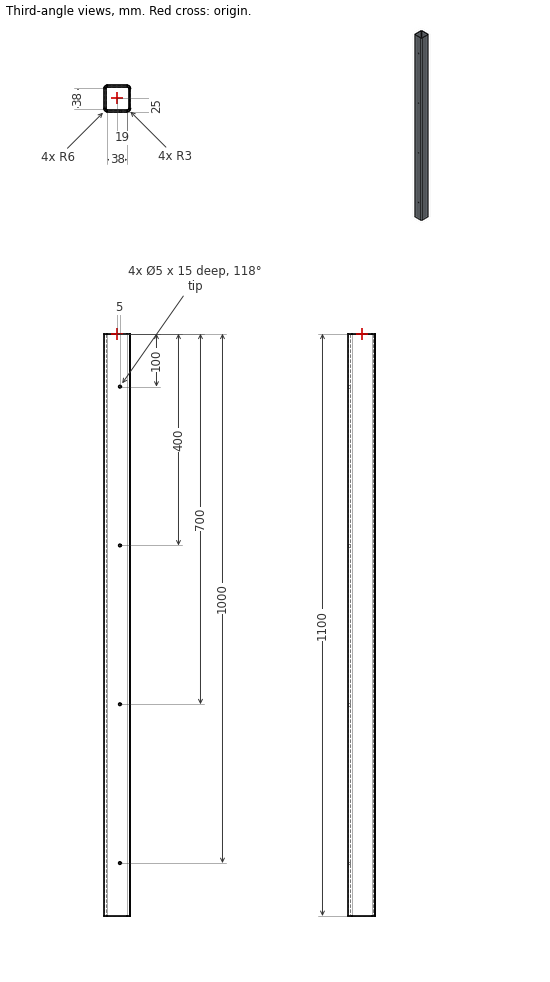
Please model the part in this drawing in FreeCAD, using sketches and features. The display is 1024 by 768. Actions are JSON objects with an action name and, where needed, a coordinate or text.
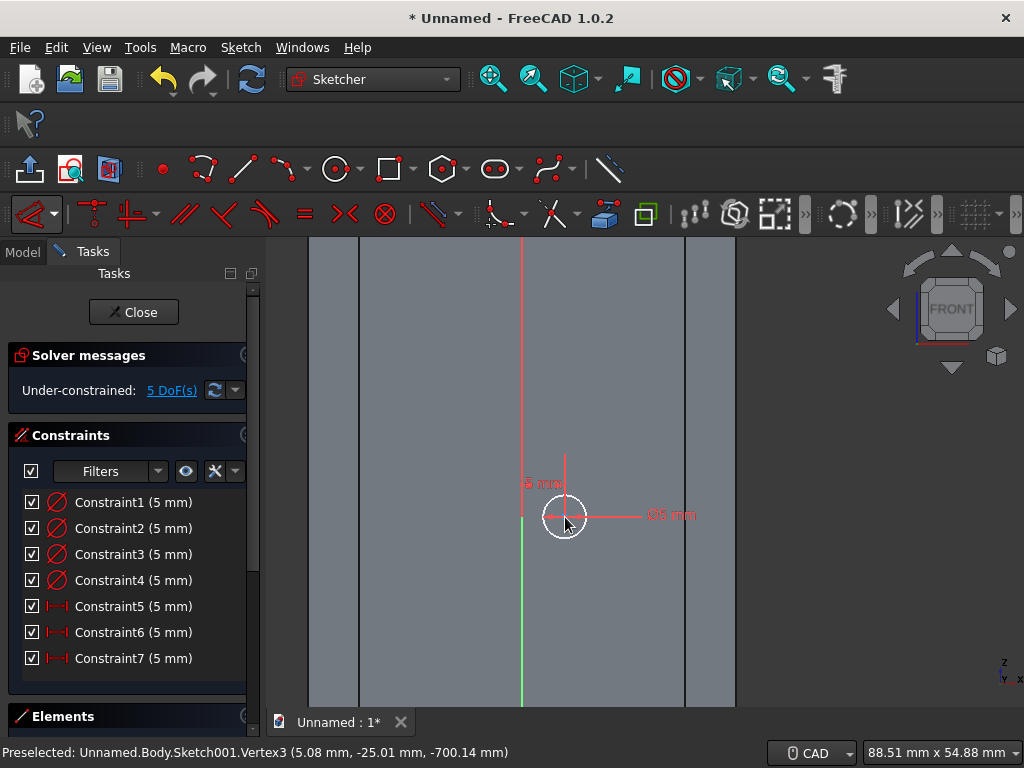
{"action": "scroll", "coordinate": [577, 542], "scroll_direction": "down", "scroll_amount": 16}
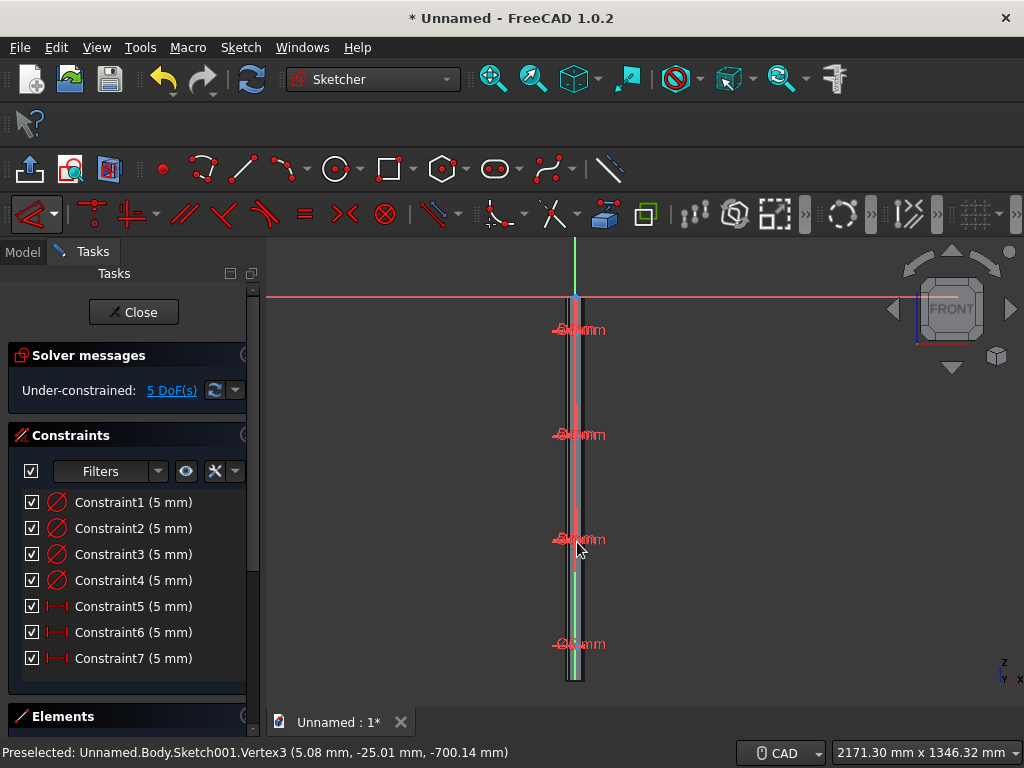
{"action": "scroll", "coordinate": [577, 646], "scroll_direction": "up", "scroll_amount": 16}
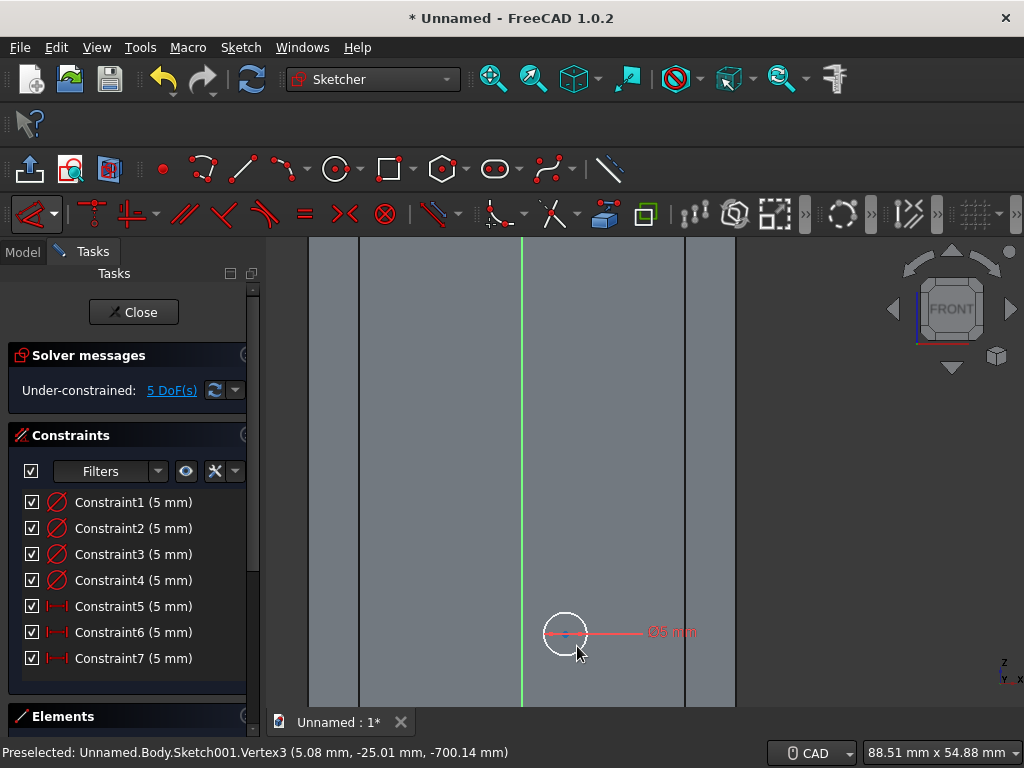
{"action": "left_click", "coordinate": [565, 634]}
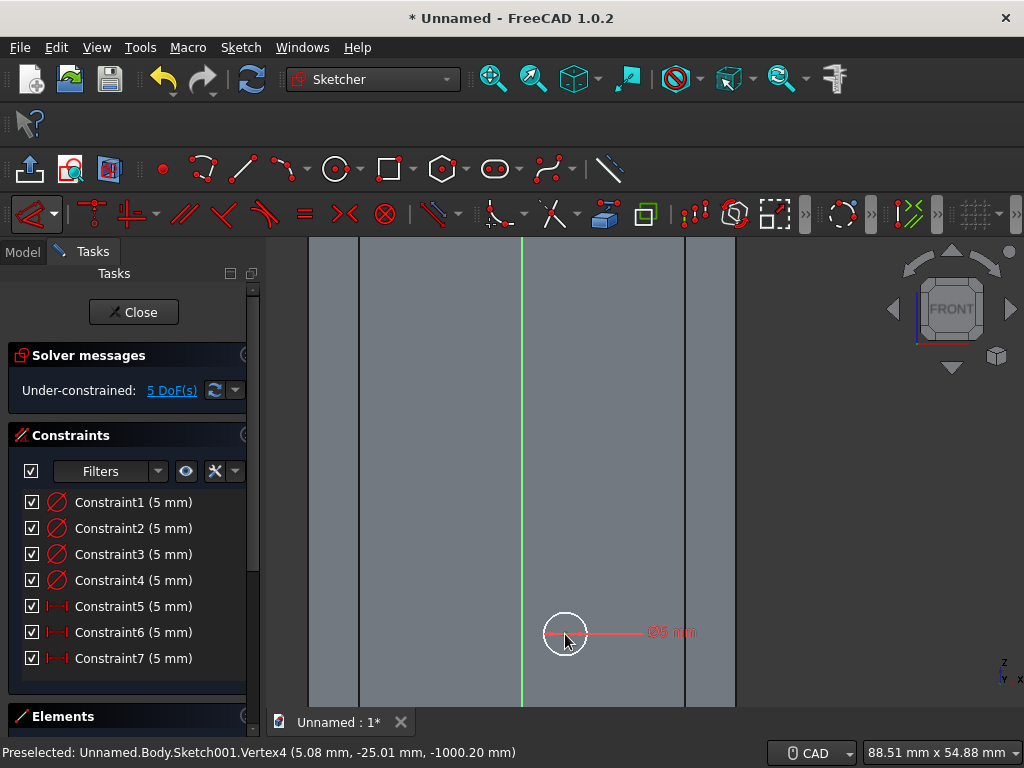
{"action": "key", "text": "l"}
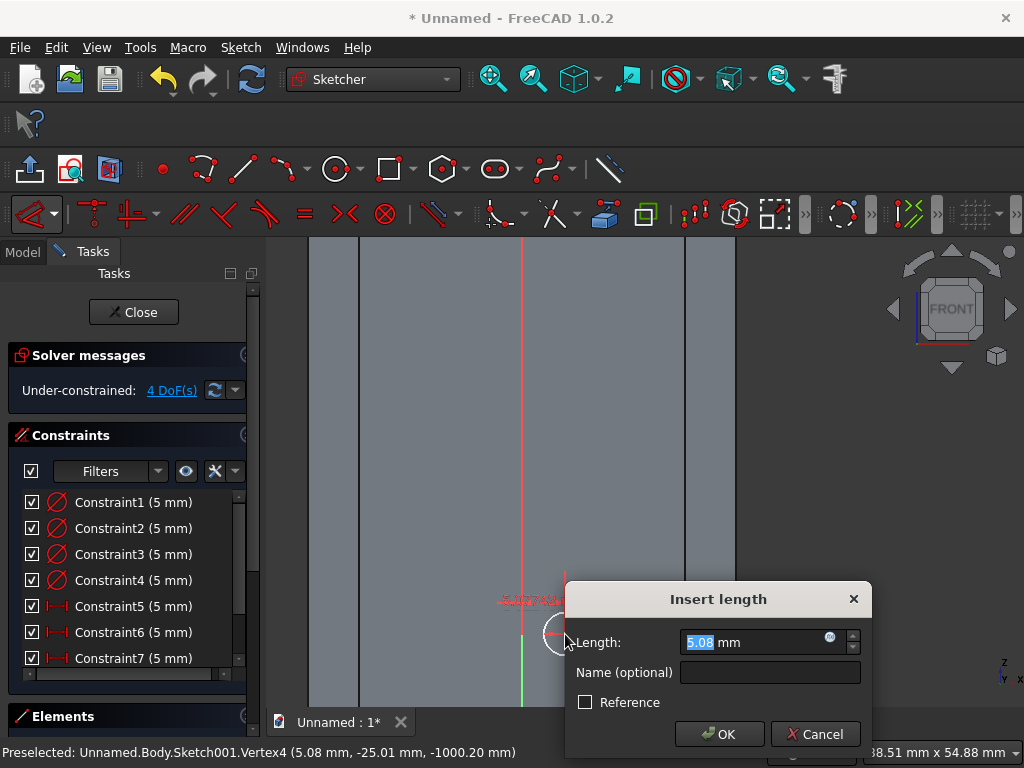
{"action": "type", "text": "5"}
{"action": "key", "text": "Return"}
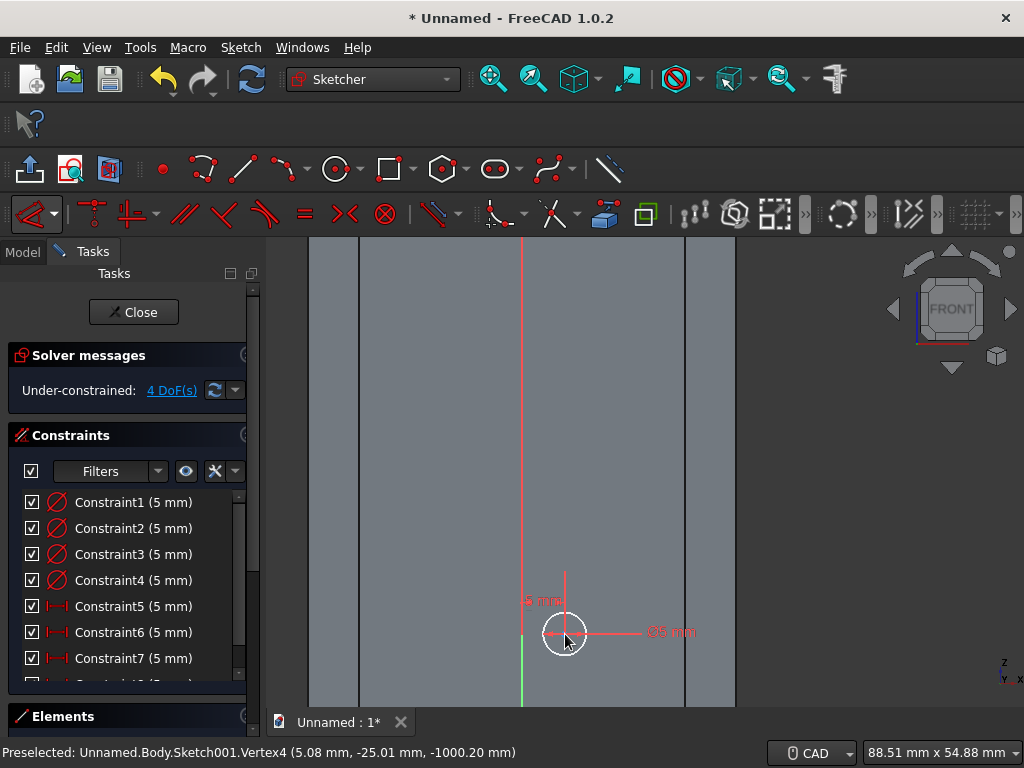
{"action": "scroll", "coordinate": [577, 647], "scroll_direction": "down", "scroll_amount": 16}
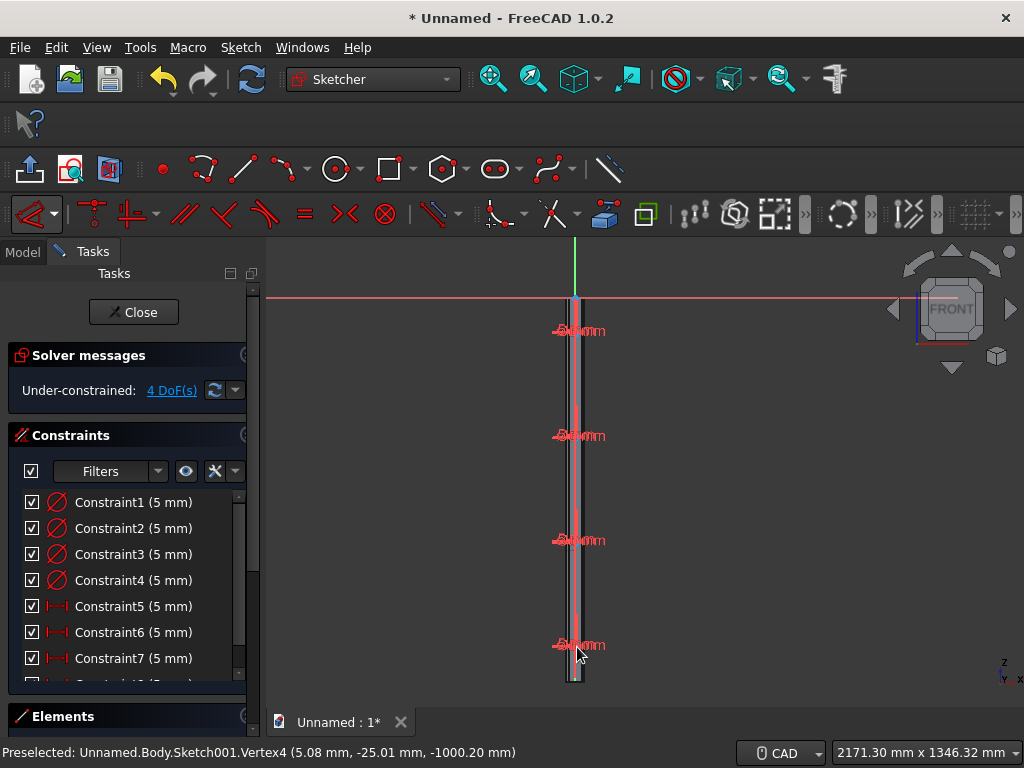
{"action": "left_click", "coordinate": [577, 333]}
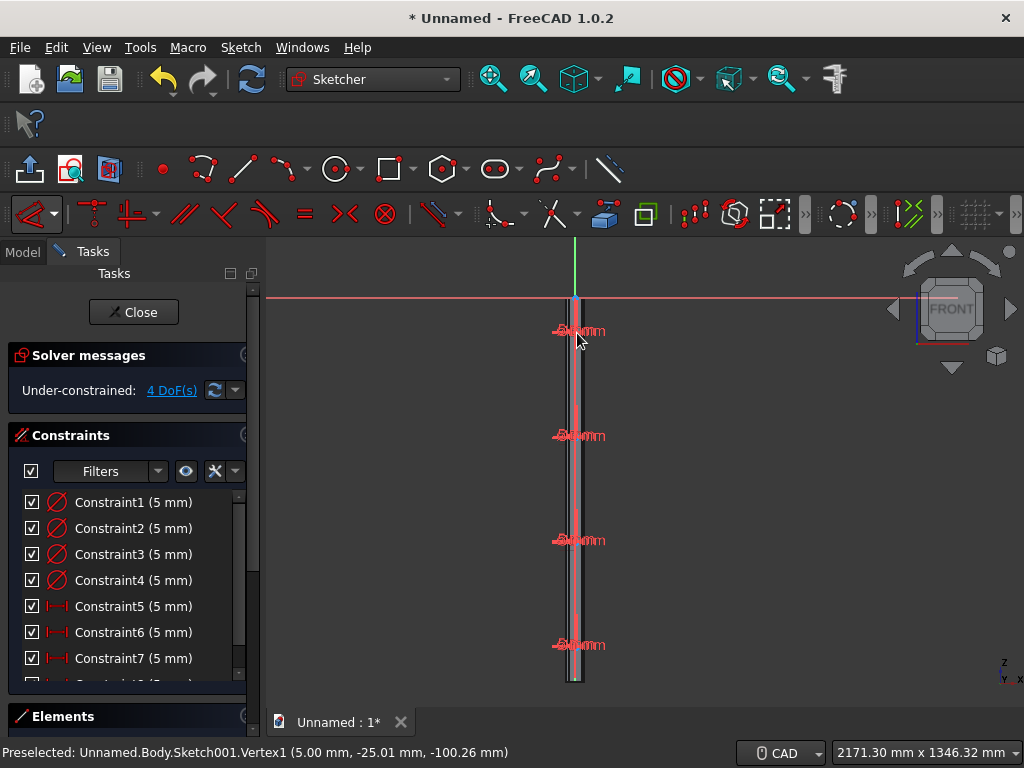
{"action": "key", "text": "i"}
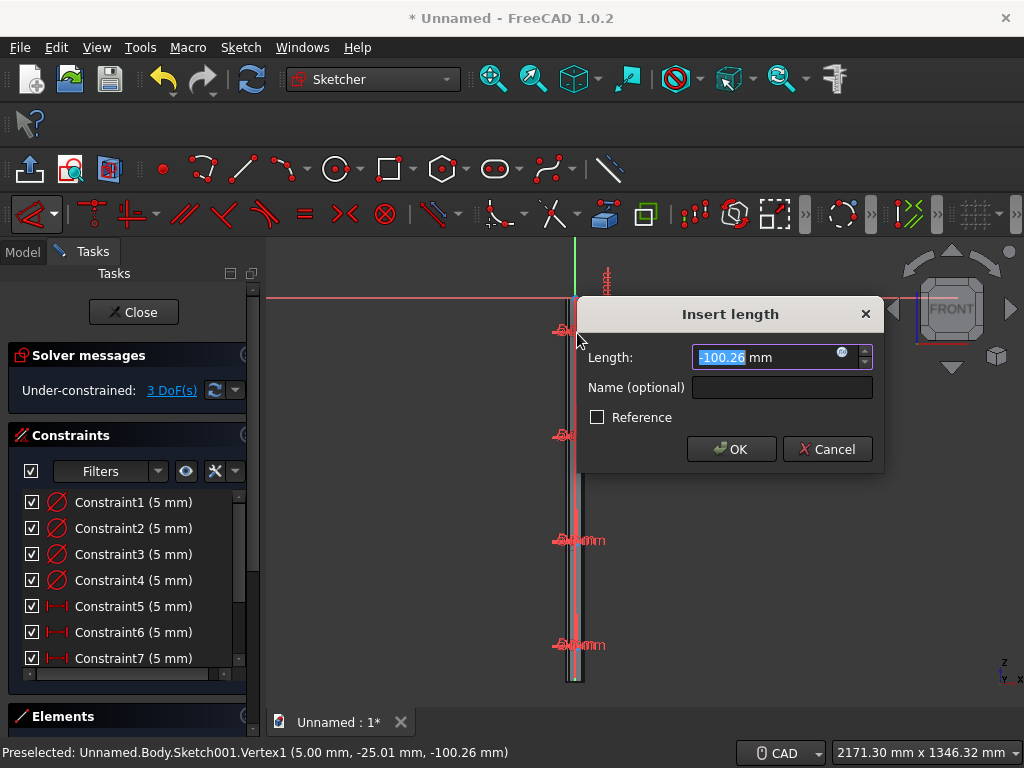
{"action": "type", "text": "-100"}
{"action": "key", "text": "Return"}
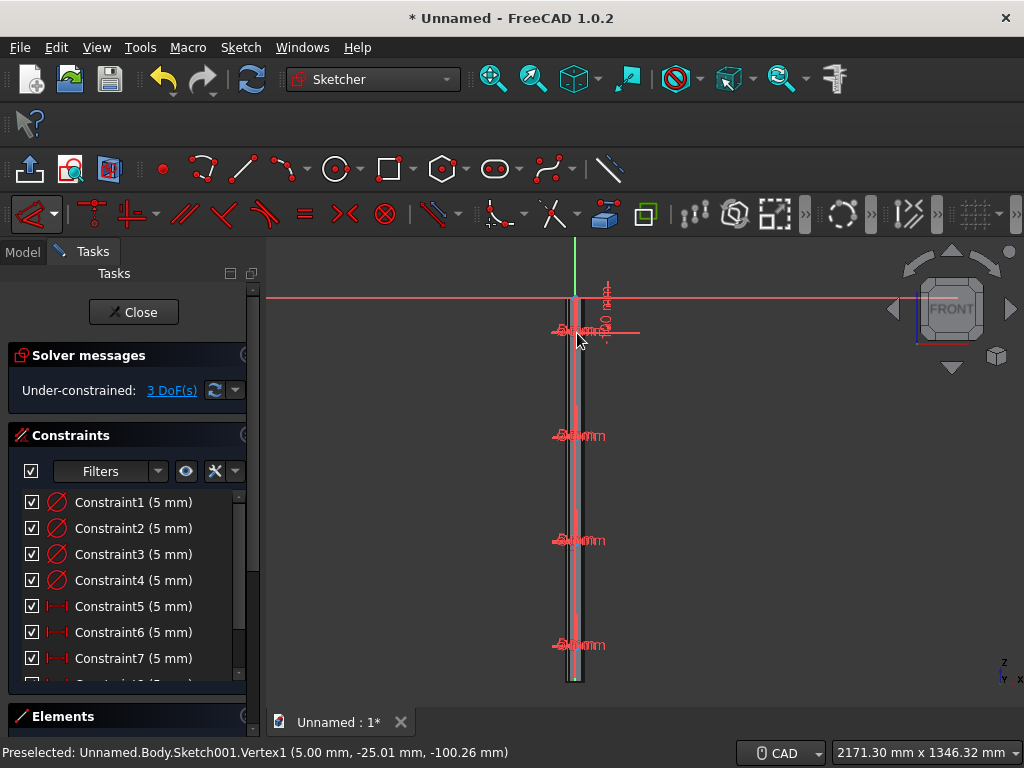
{"action": "left_click", "coordinate": [577, 438]}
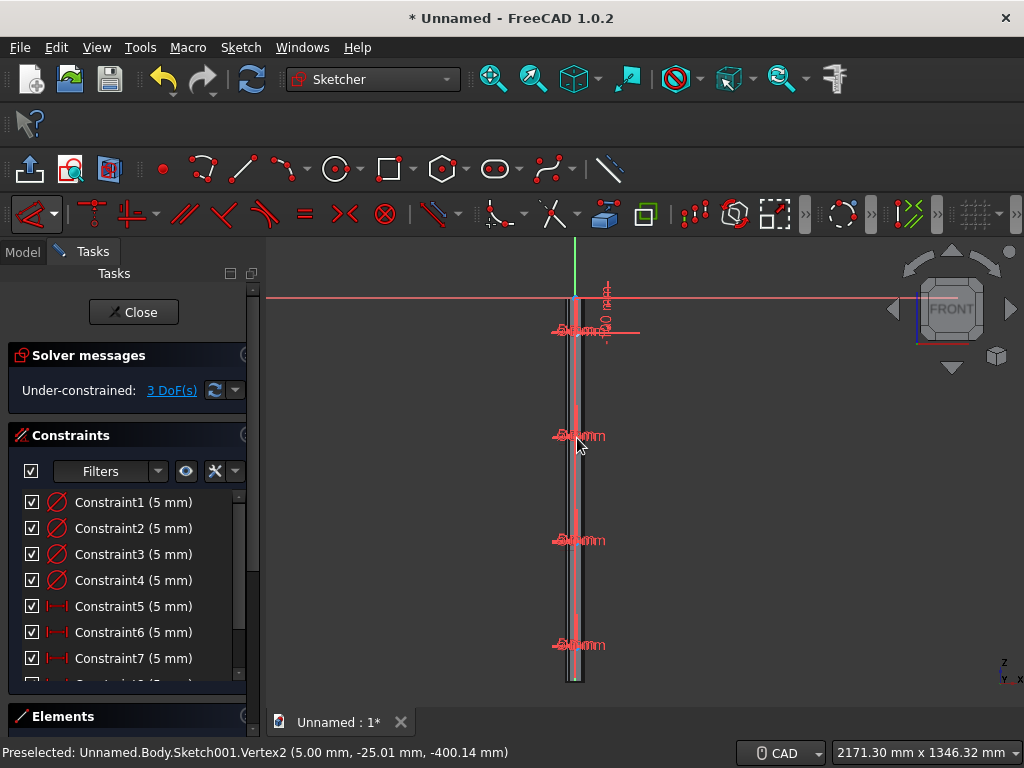
{"action": "key", "text": "i"}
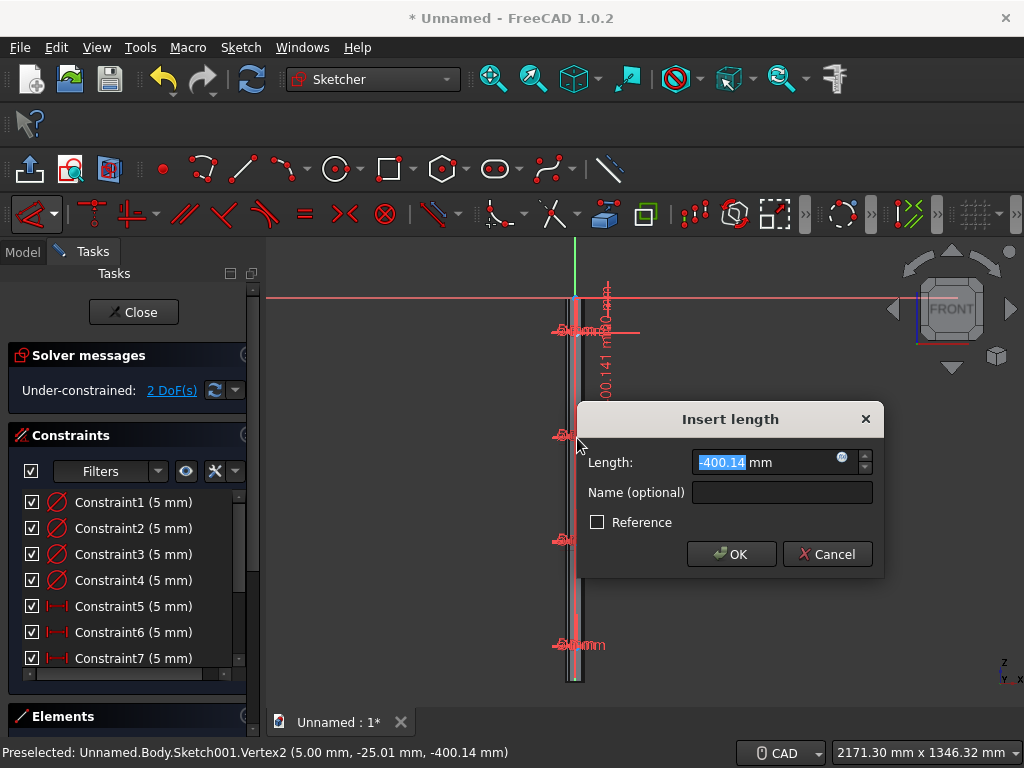
{"action": "type", "text": "-400"}
{"action": "key", "text": "Return"}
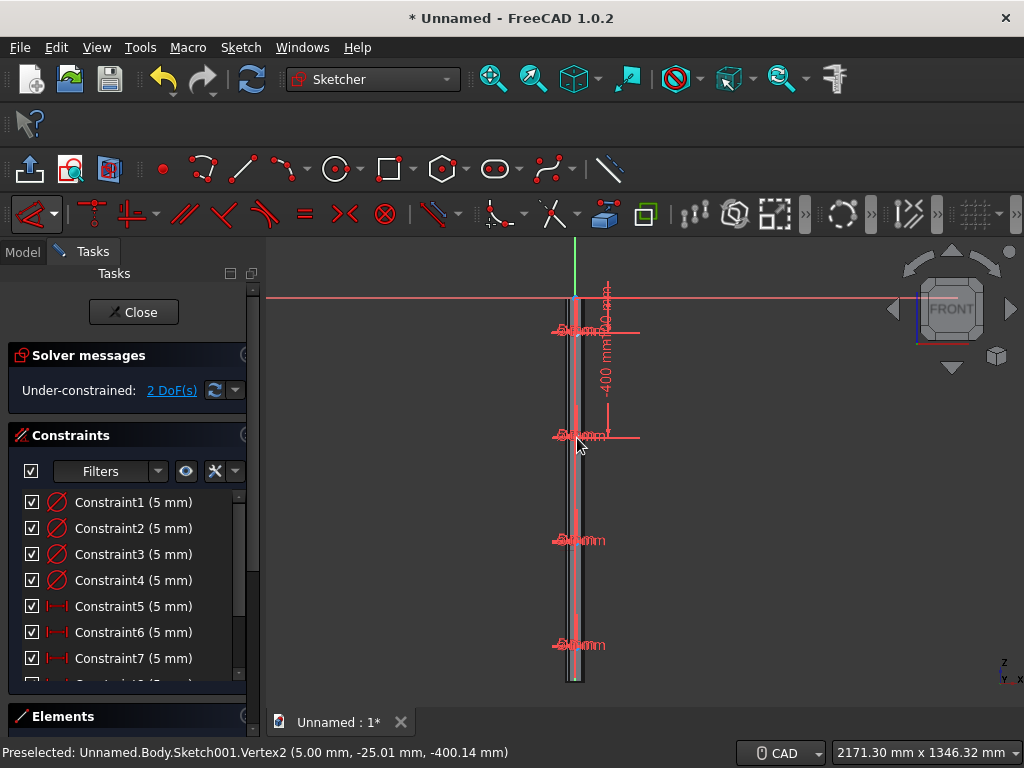
{"action": "left_click", "coordinate": [577, 543]}